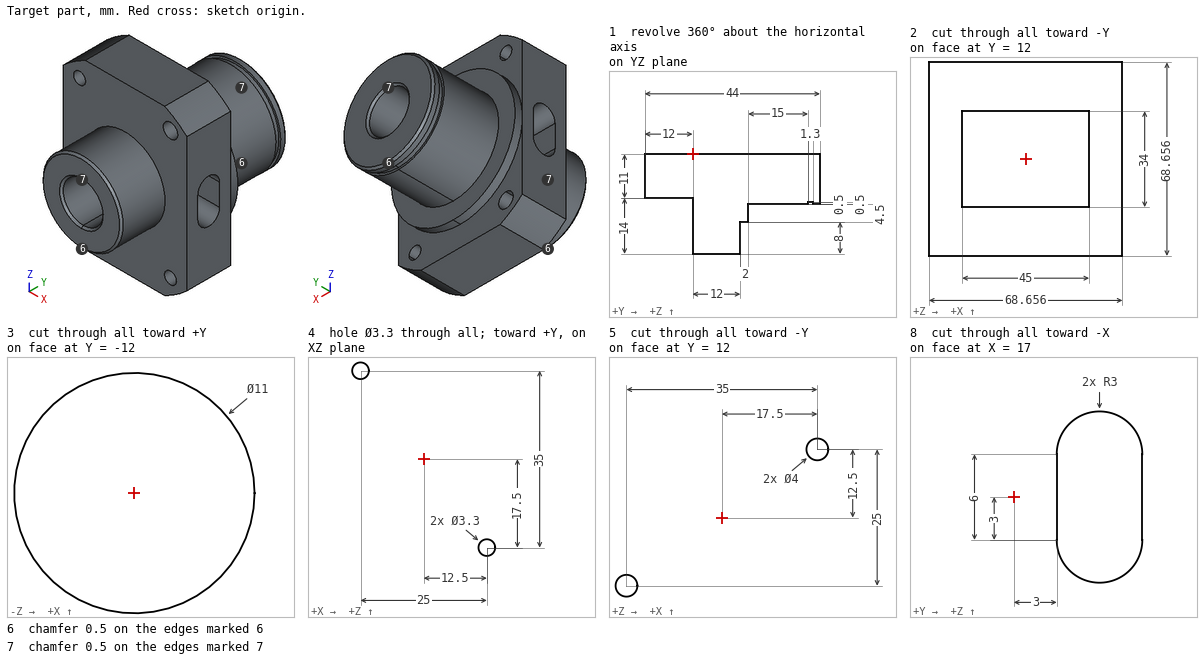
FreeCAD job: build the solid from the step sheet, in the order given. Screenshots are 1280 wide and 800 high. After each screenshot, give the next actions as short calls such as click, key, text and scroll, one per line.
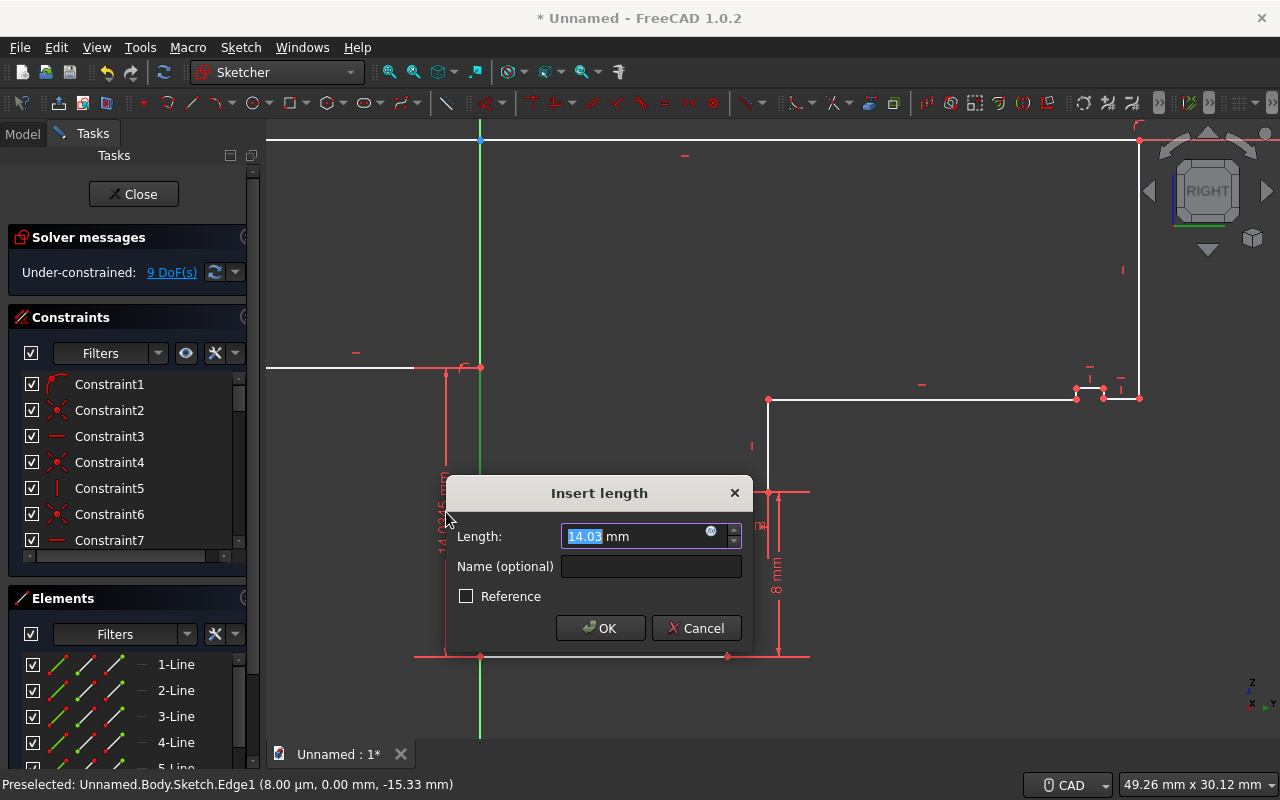
text(14)
key(Return)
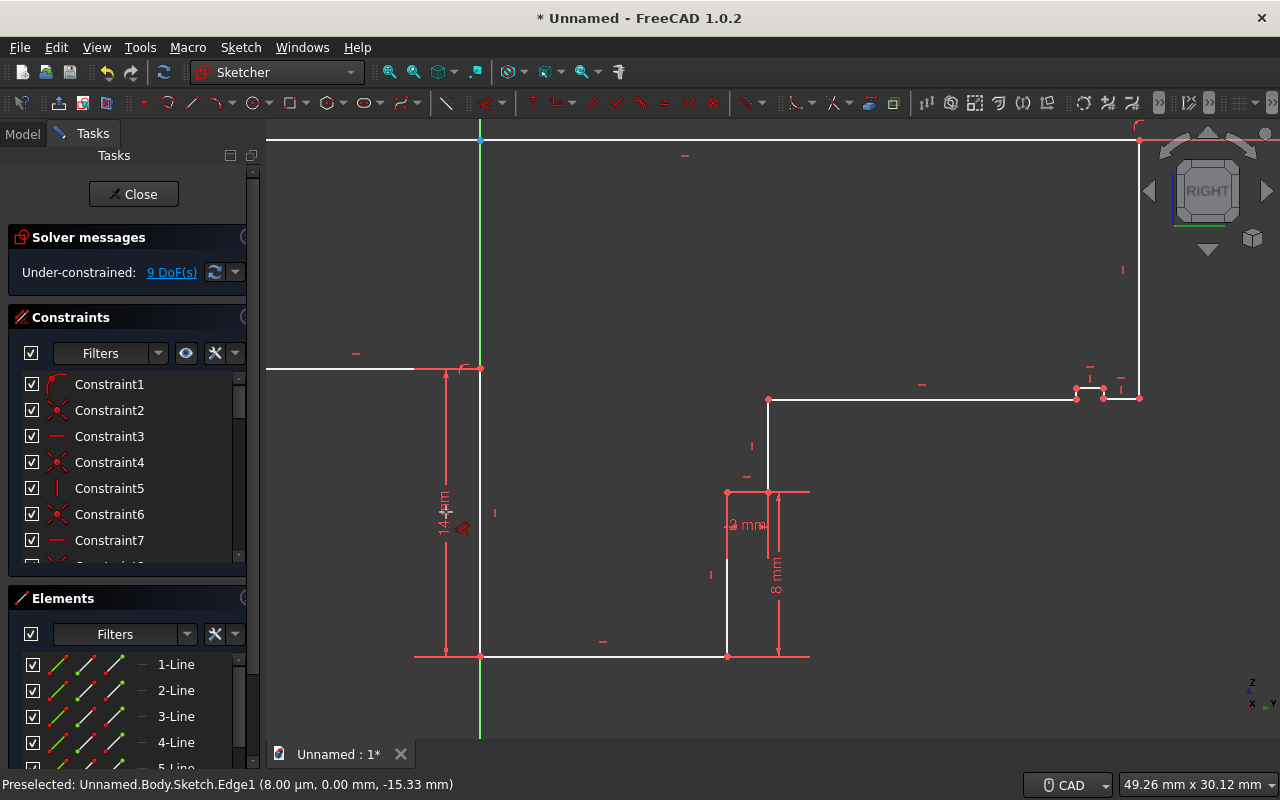
click(554, 657)
click(604, 691)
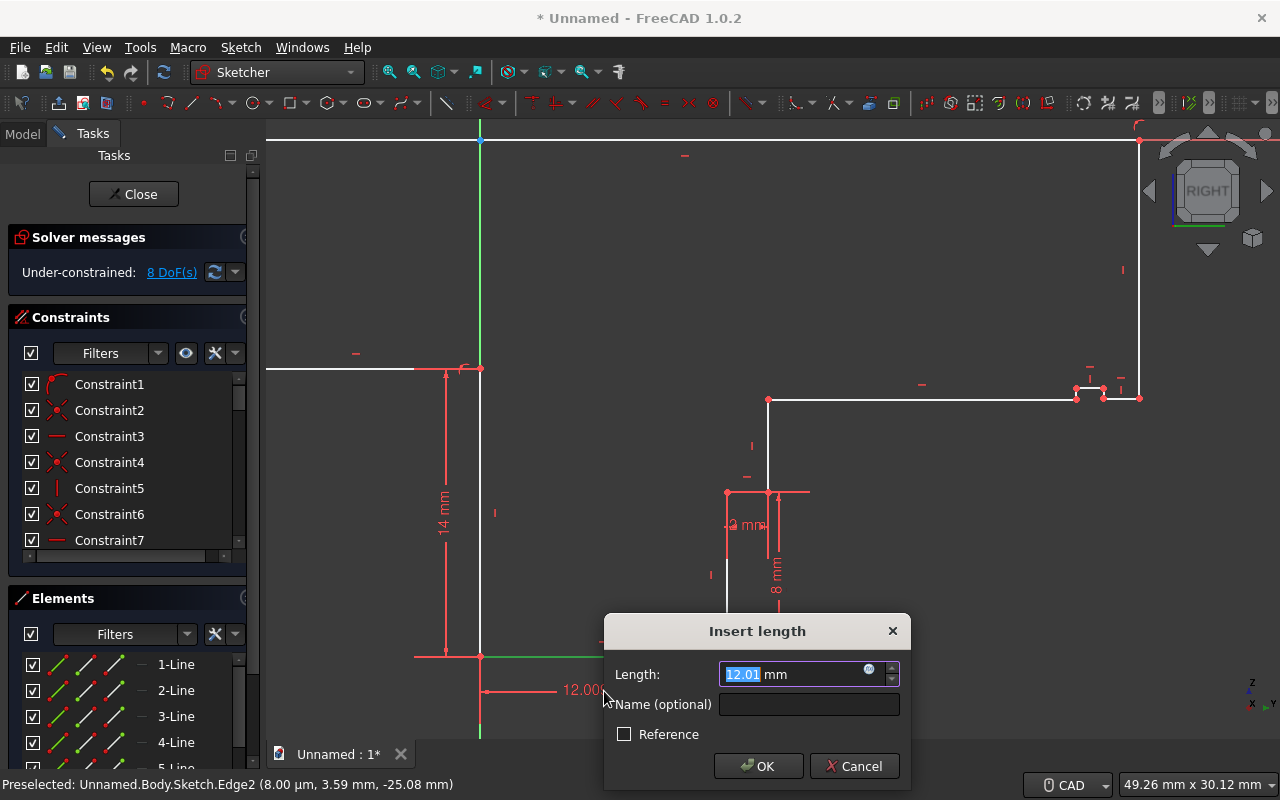
text(12)
key(Return)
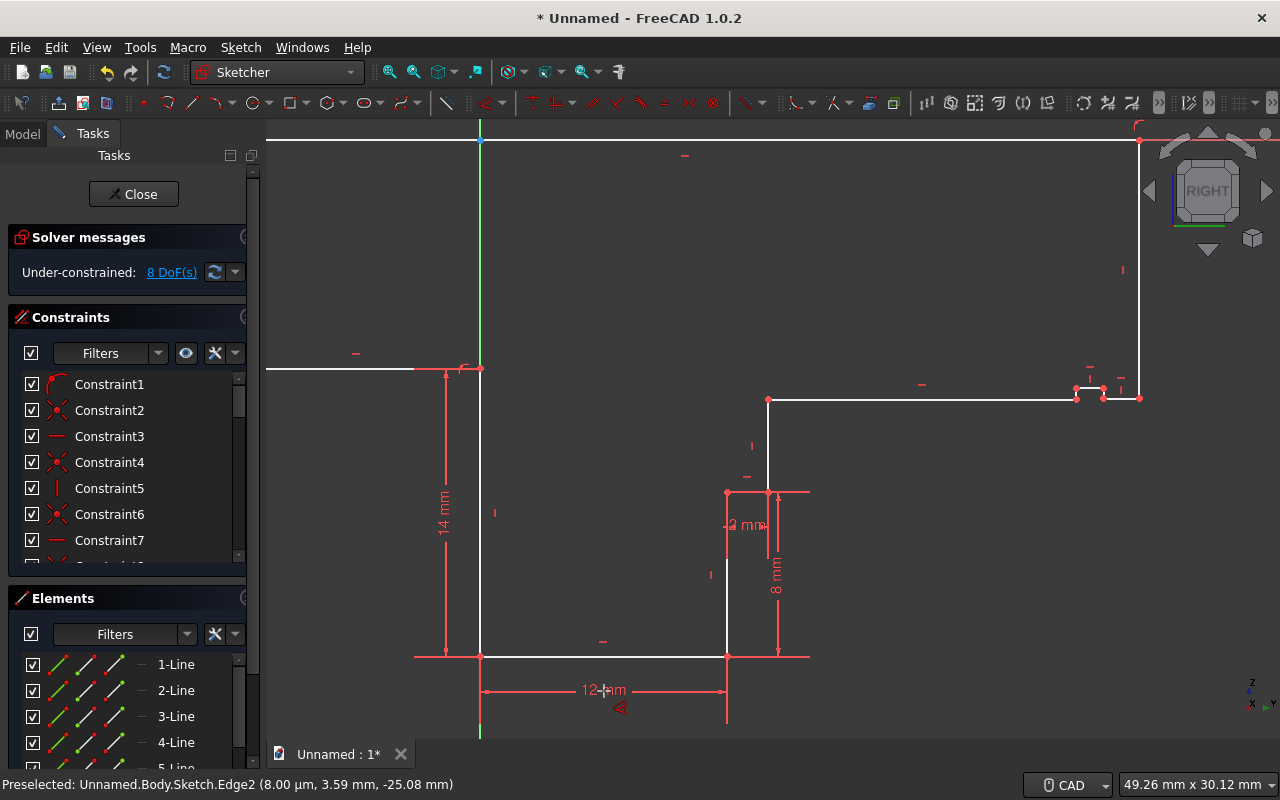
click(861, 400)
click(922, 434)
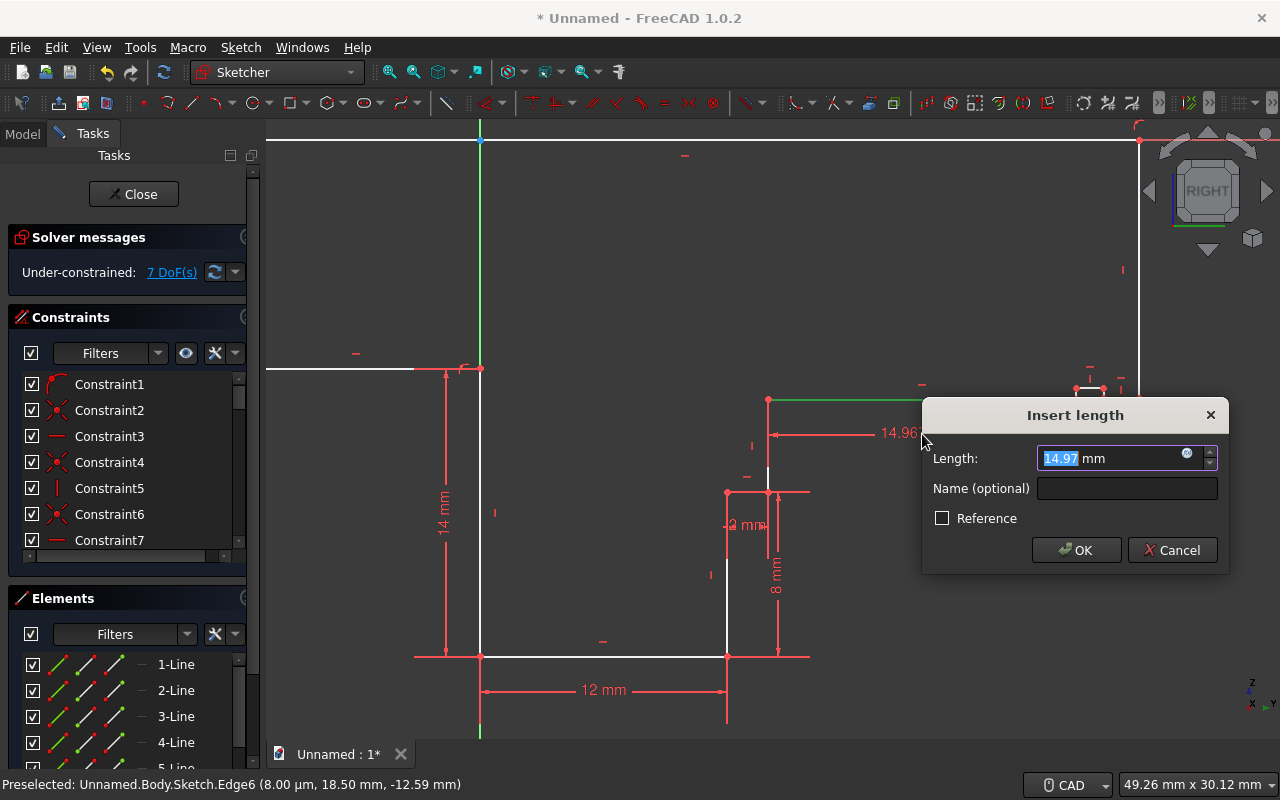
text(15)
key(Return)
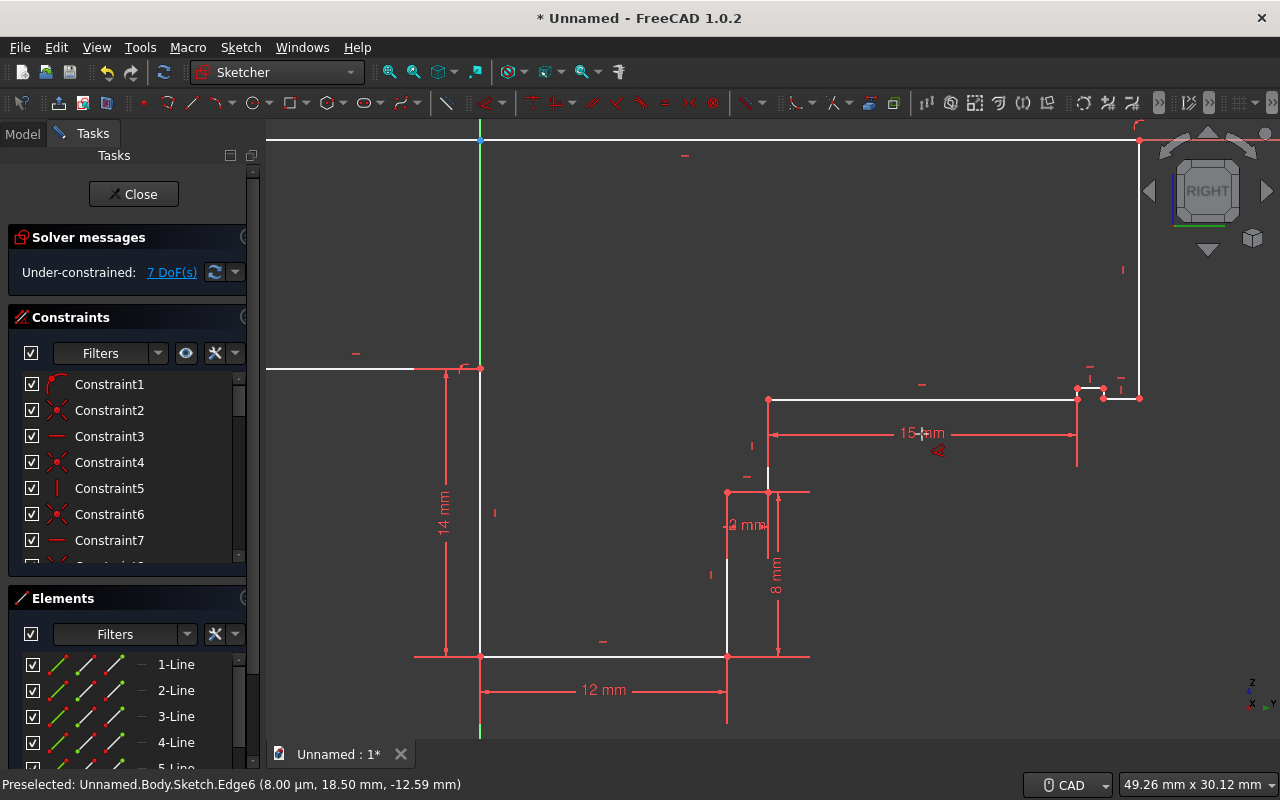
scroll(742, 492, down, 2)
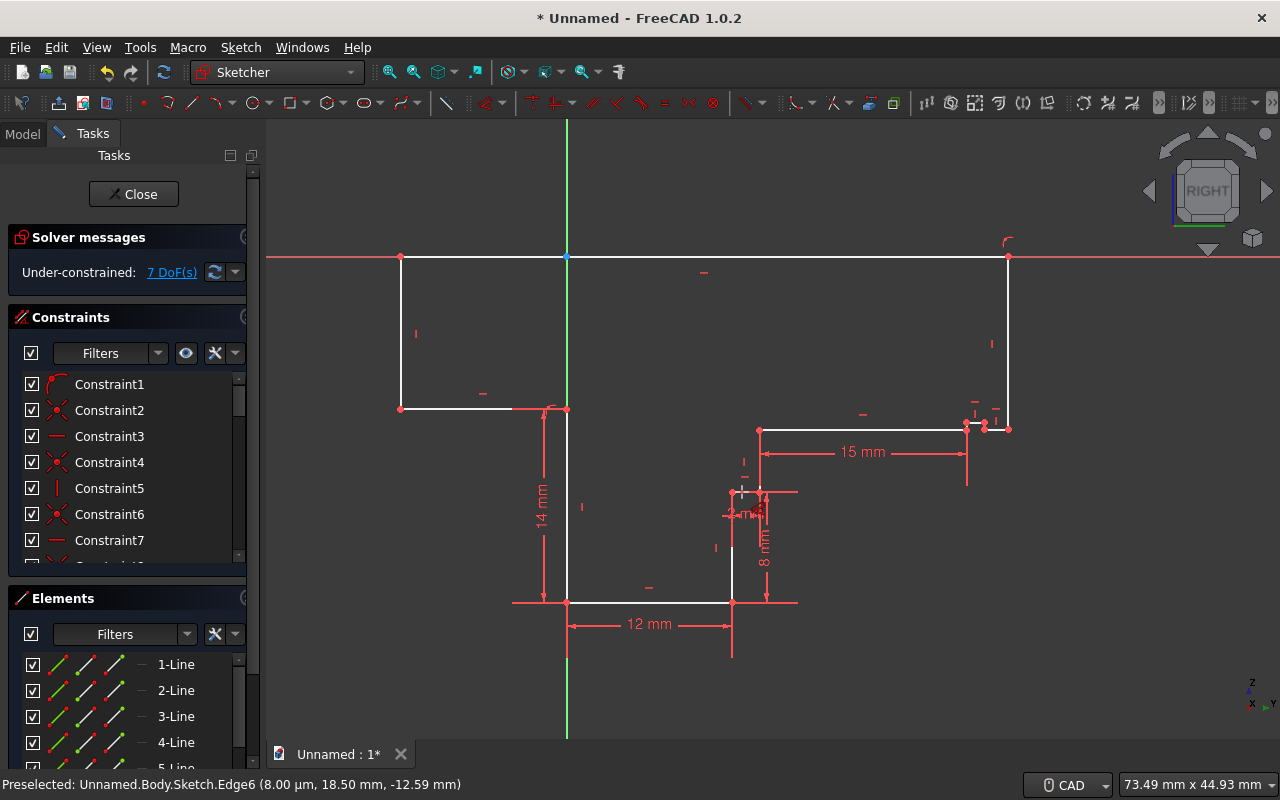
click(826, 257)
click(704, 223)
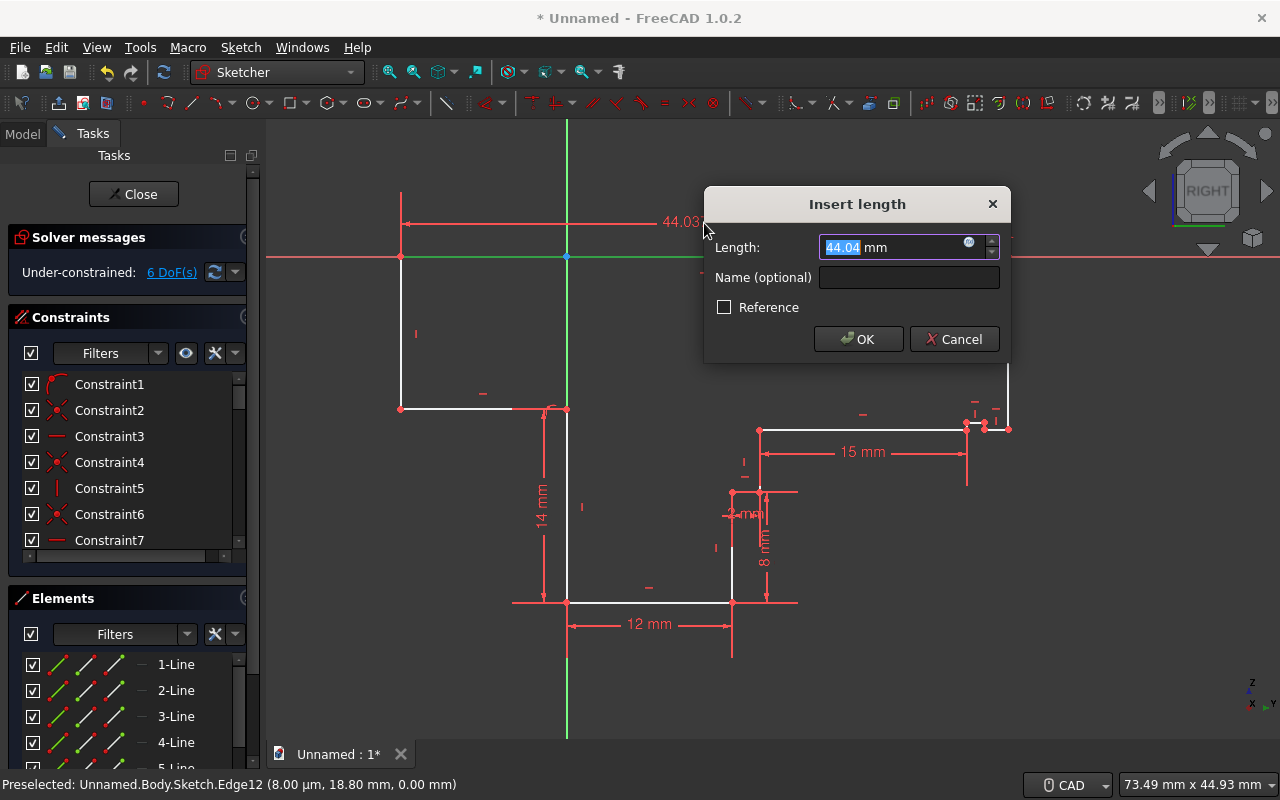
text(44)
key(Return)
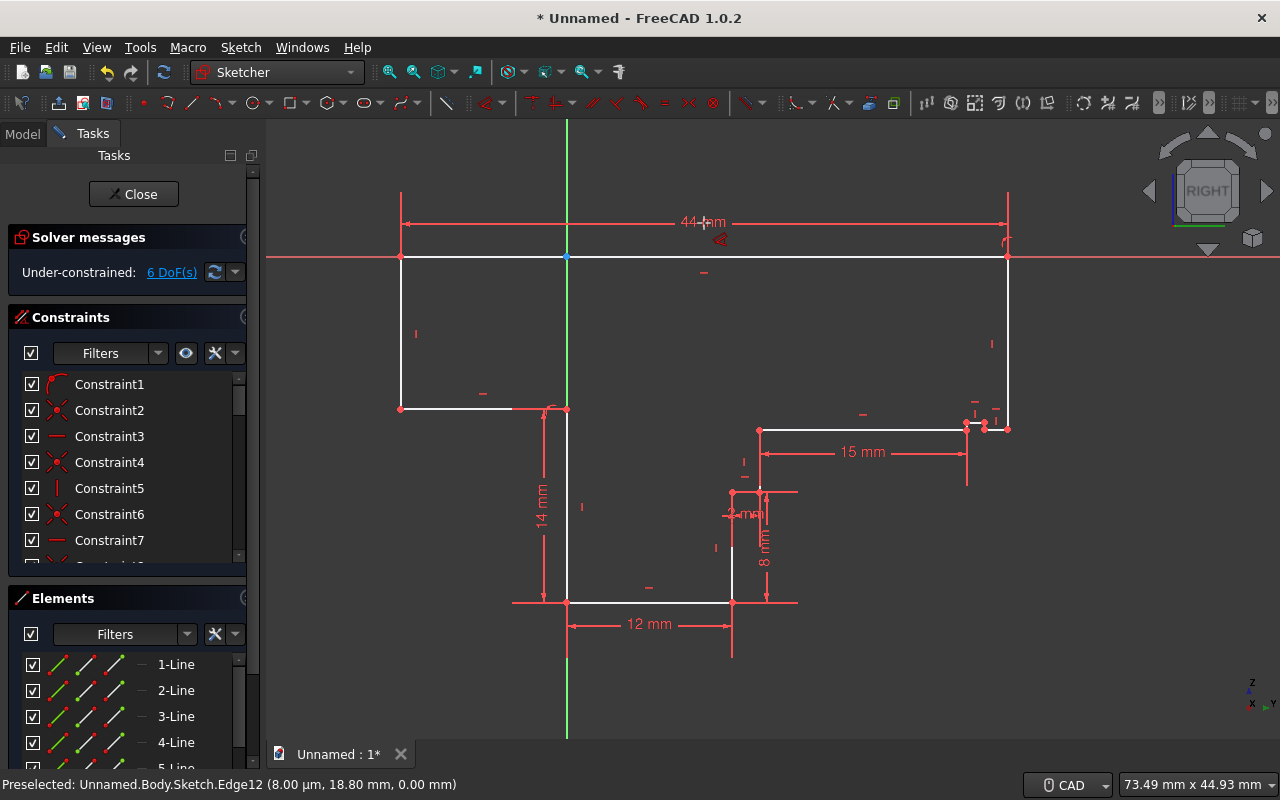
click(401, 302)
click(367, 333)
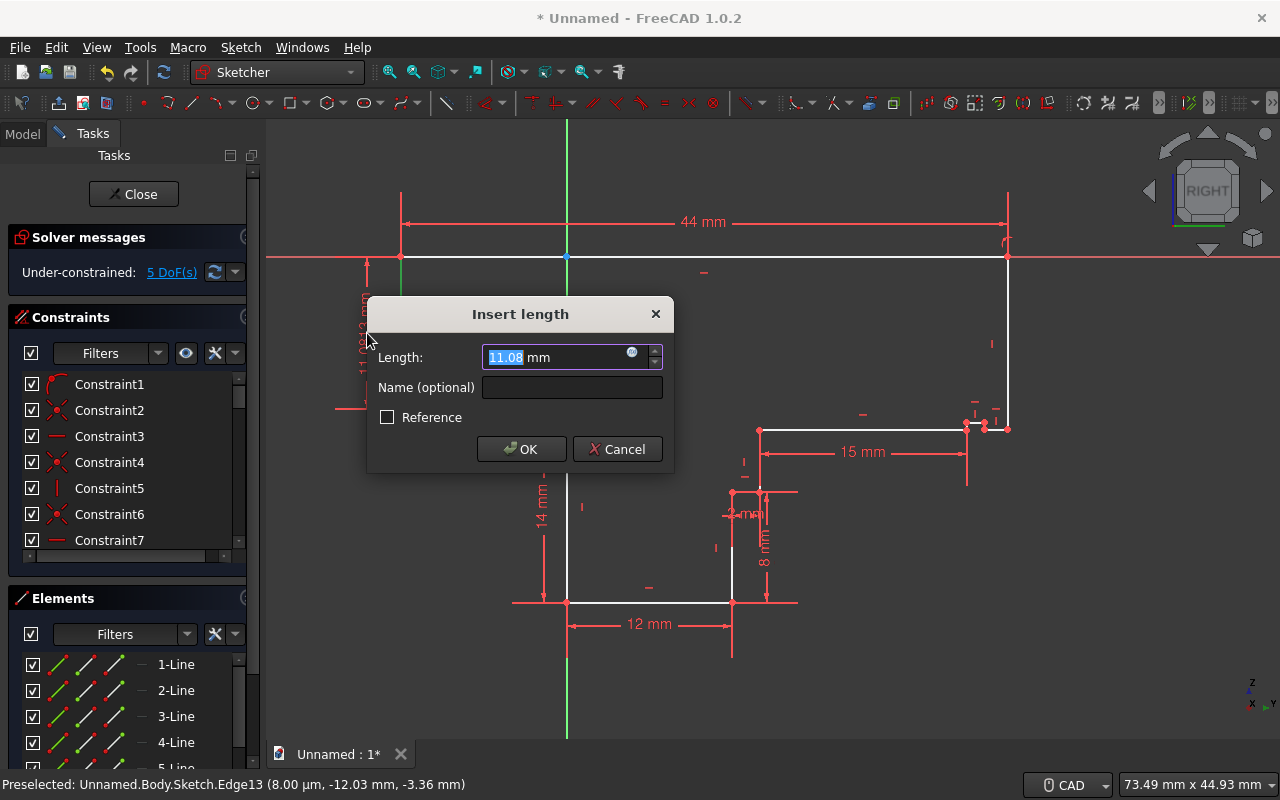
text(11)
key(Return)